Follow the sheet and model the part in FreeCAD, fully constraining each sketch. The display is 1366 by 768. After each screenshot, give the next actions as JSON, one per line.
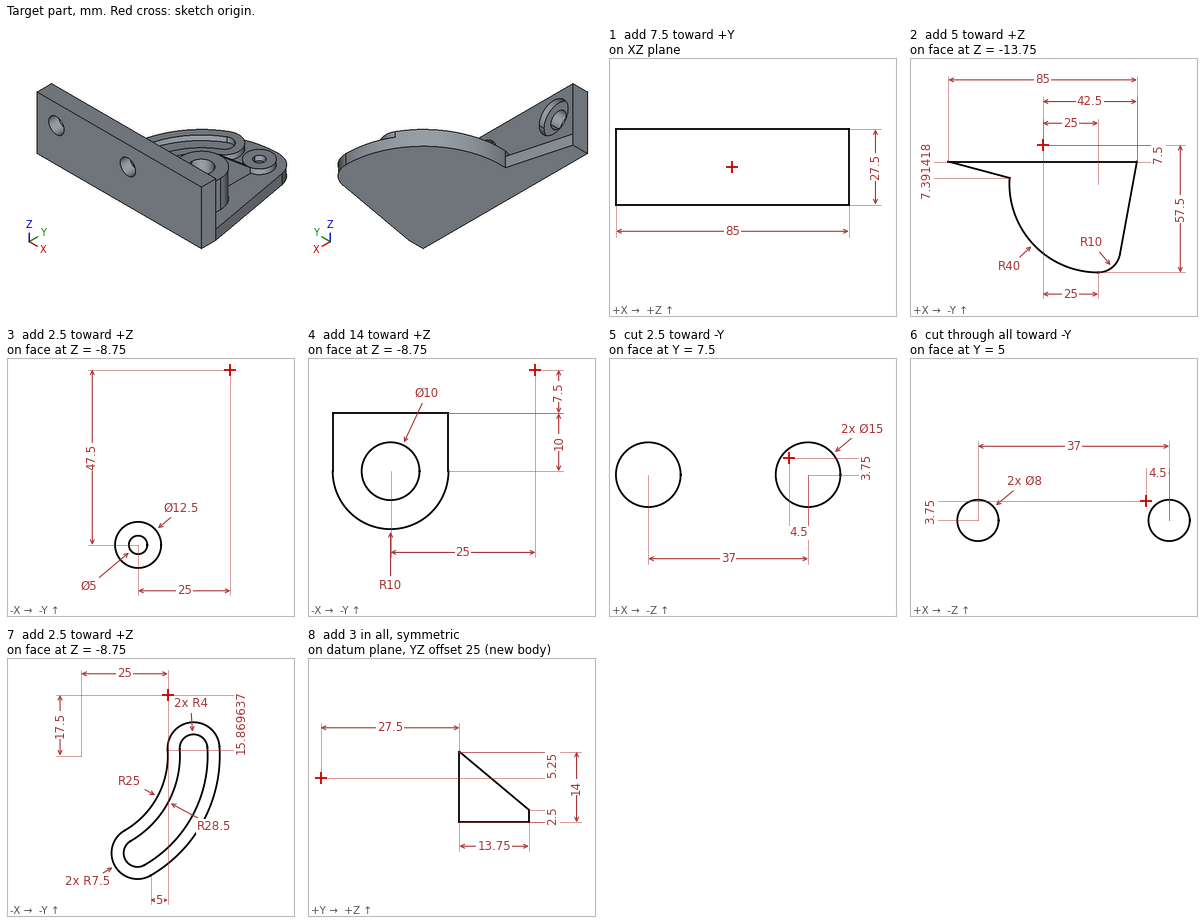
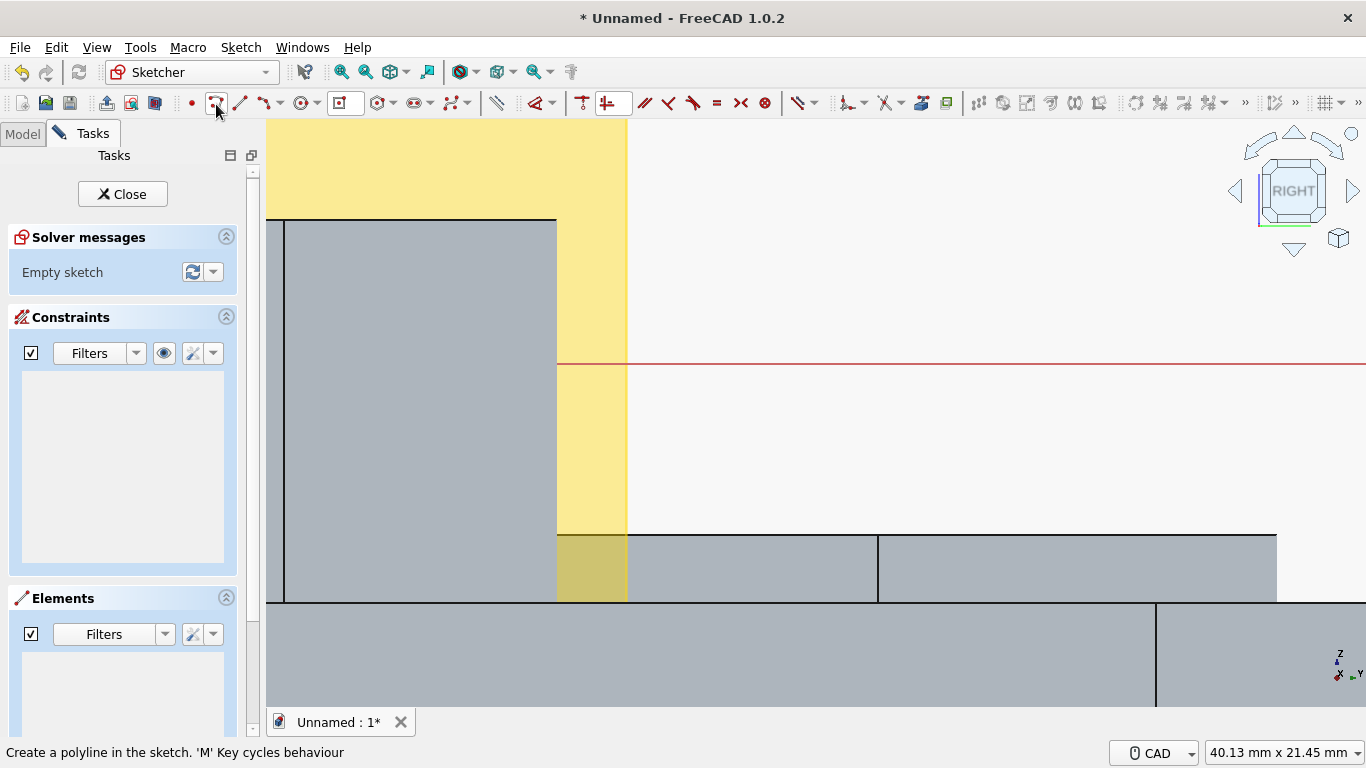
{"action": "left_click", "coordinate": [558, 220]}
{"action": "left_click", "coordinate": [558, 603]}
{"action": "left_click", "coordinate": [935, 603]}
{"action": "left_click", "coordinate": [935, 535]}
{"action": "left_click", "coordinate": [558, 221]}
{"action": "key", "text": "Escape"}
{"action": "key", "text": "Escape"}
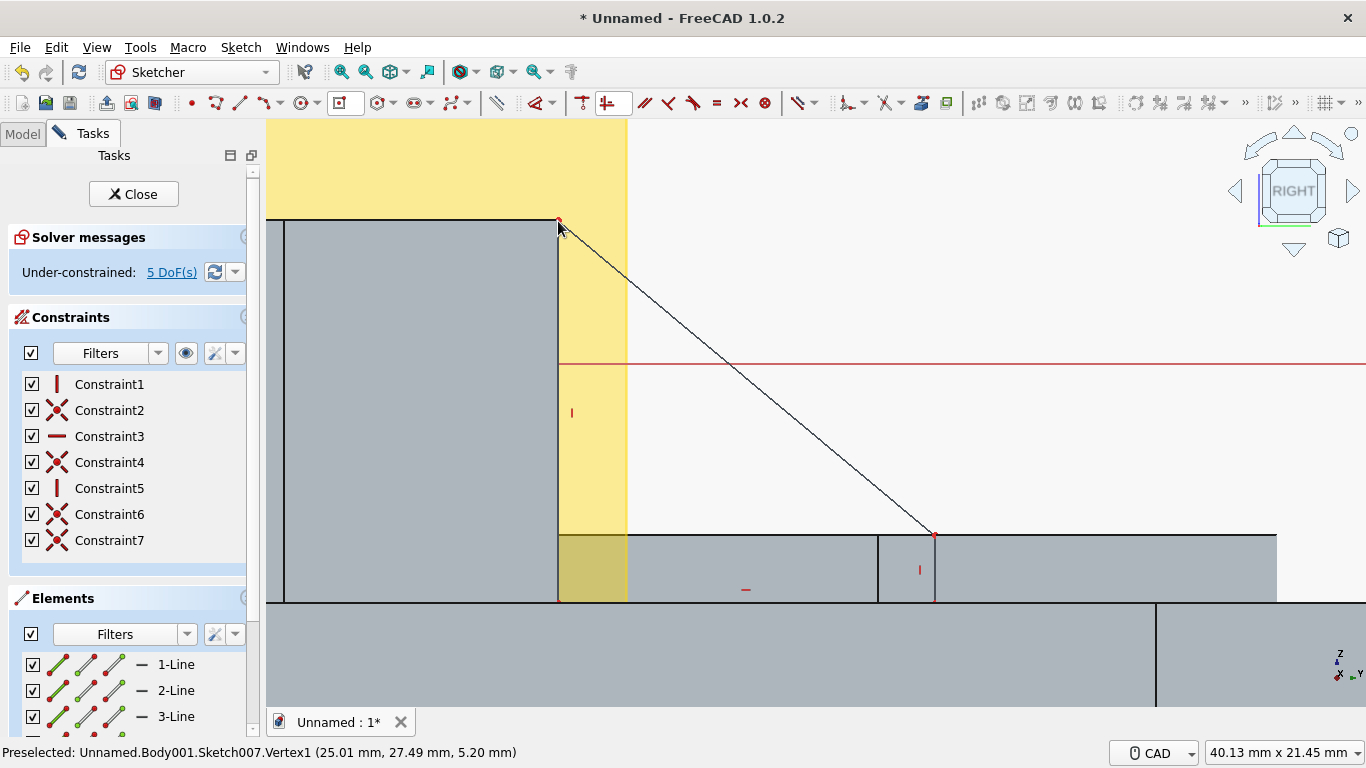
{"action": "left_click", "coordinate": [536, 104]}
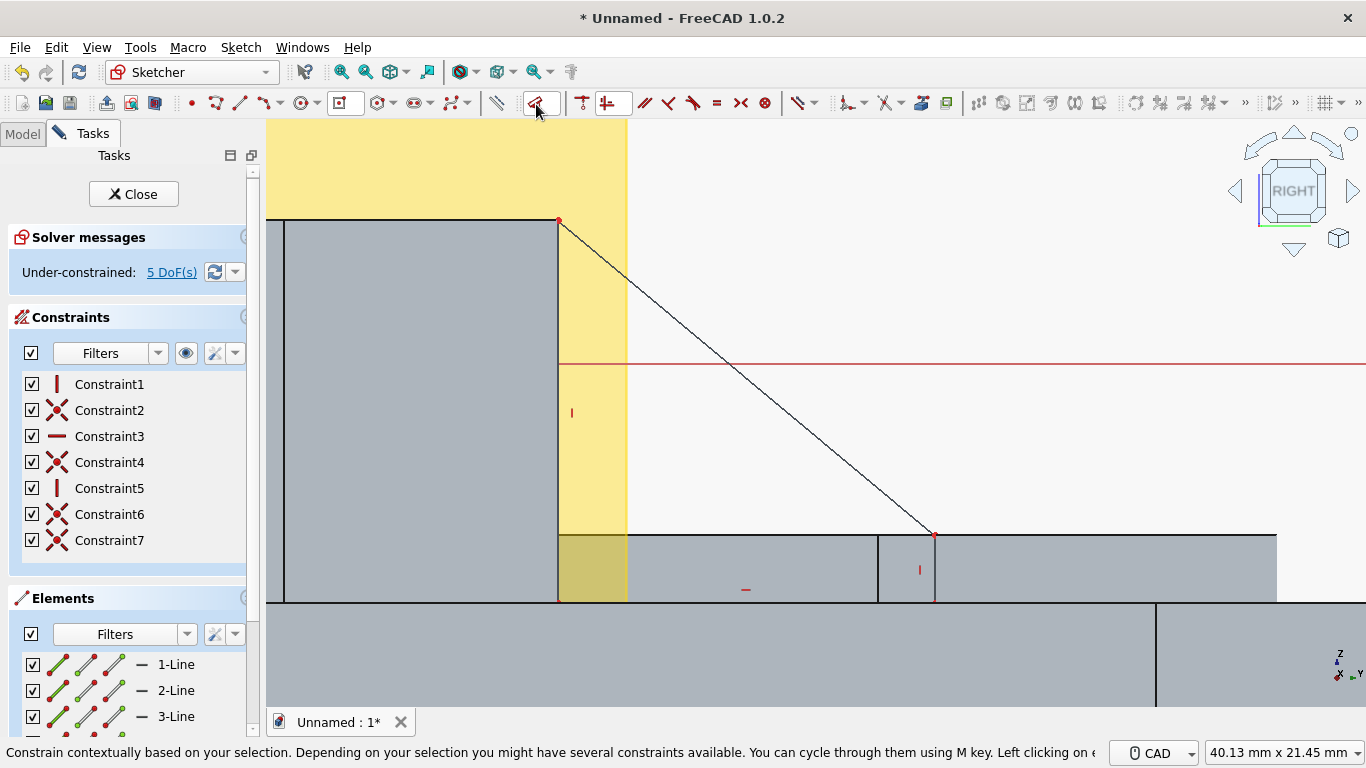
{"action": "left_click", "coordinate": [558, 336]}
{"action": "left_click", "coordinate": [524, 412]}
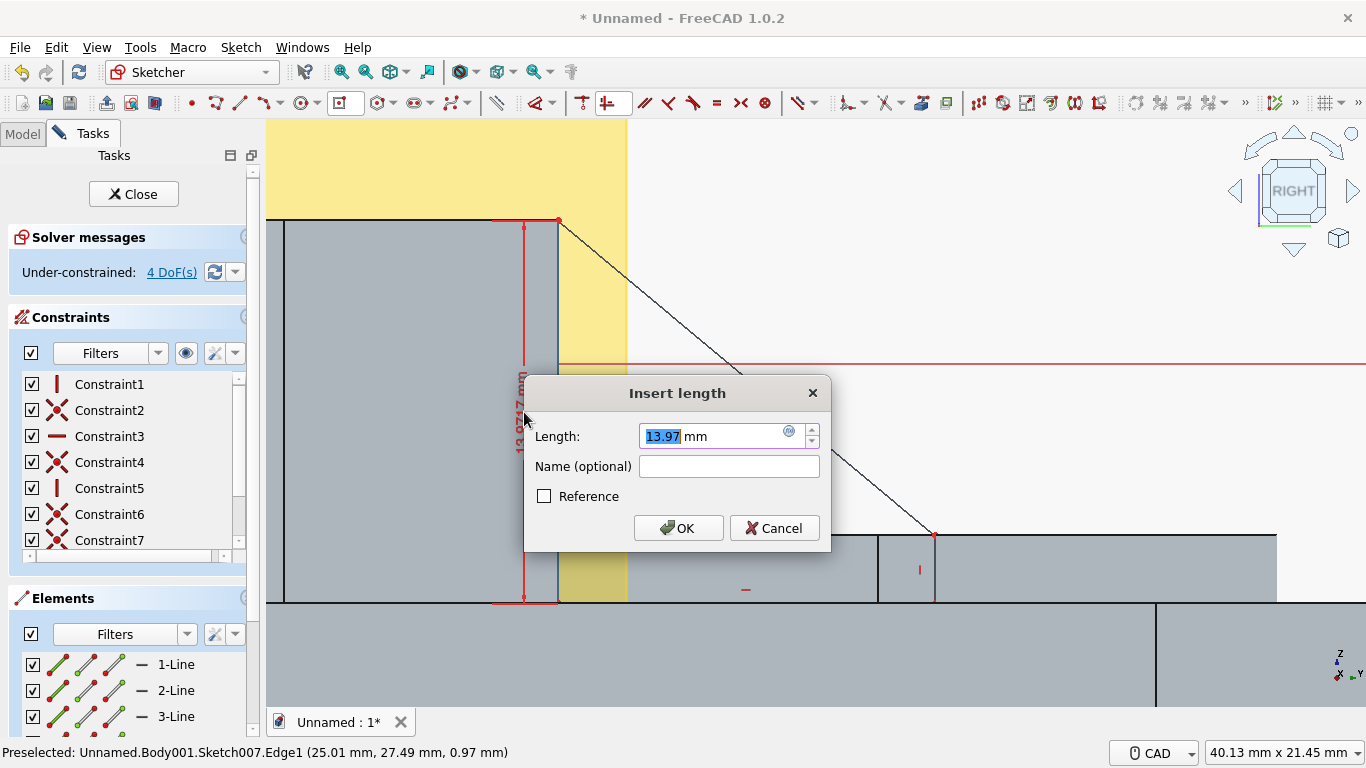
{"action": "type", "text": "14"}
{"action": "key", "text": "Return"}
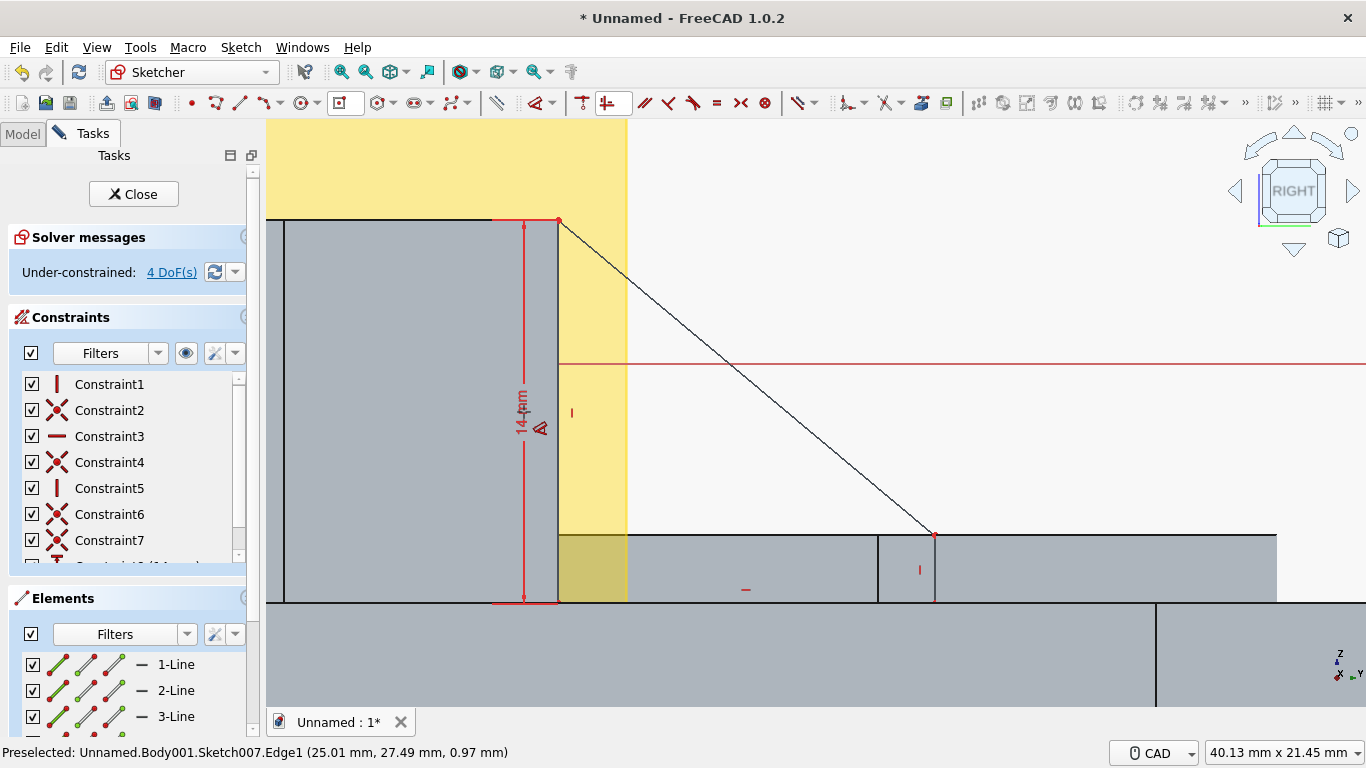
{"action": "left_click", "coordinate": [935, 584]}
{"action": "left_click", "coordinate": [969, 570]}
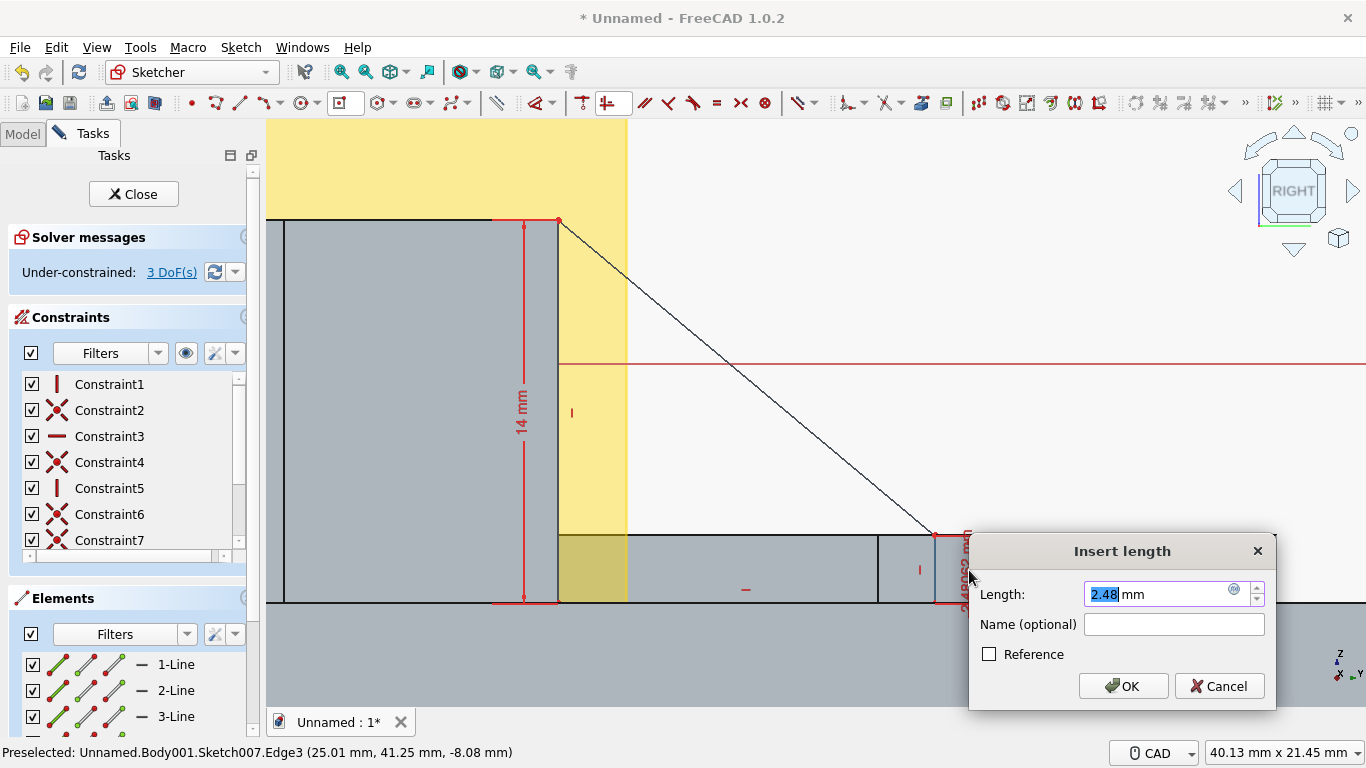
{"action": "type", "text": "2.5"}
{"action": "key", "text": "Return"}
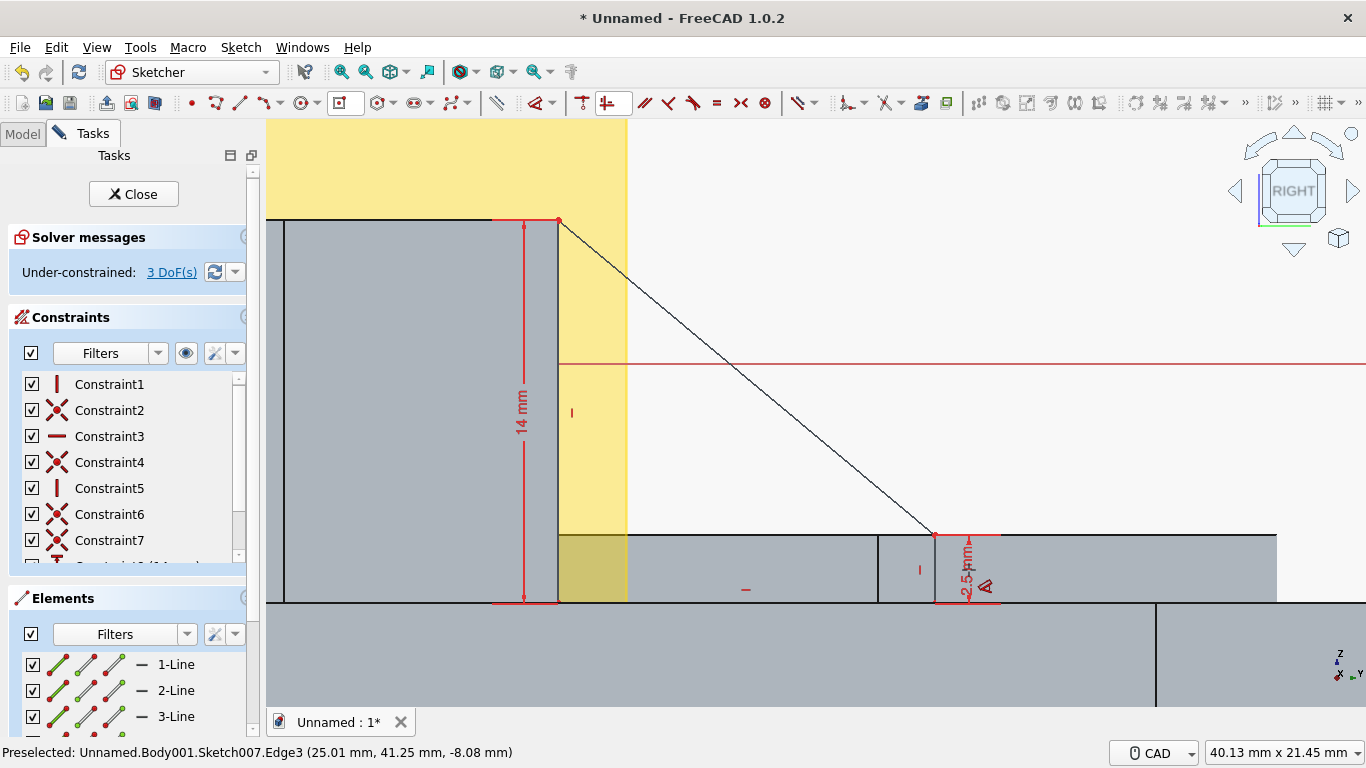
{"action": "left_click", "coordinate": [671, 604]}
{"action": "left_click", "coordinate": [747, 638]}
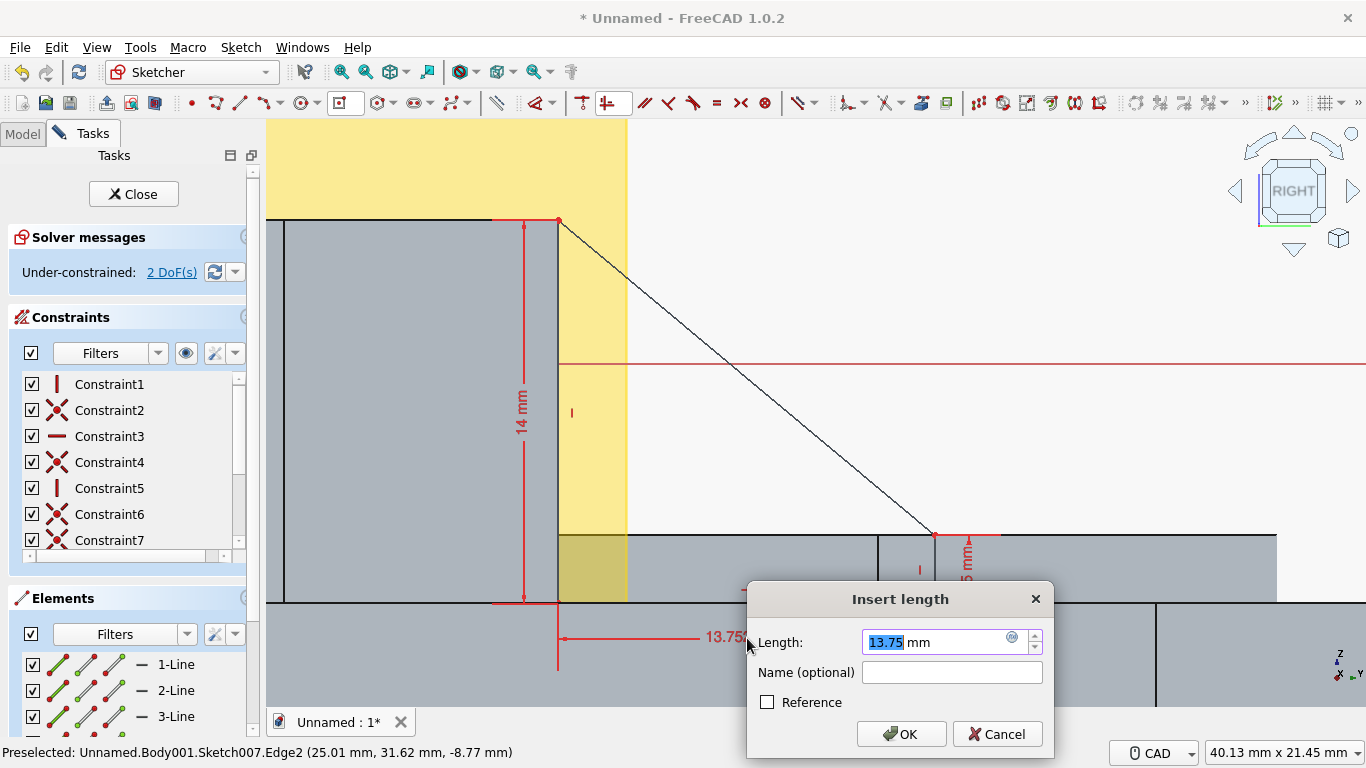
{"action": "type", "text": "13.75"}
{"action": "key", "text": "Return"}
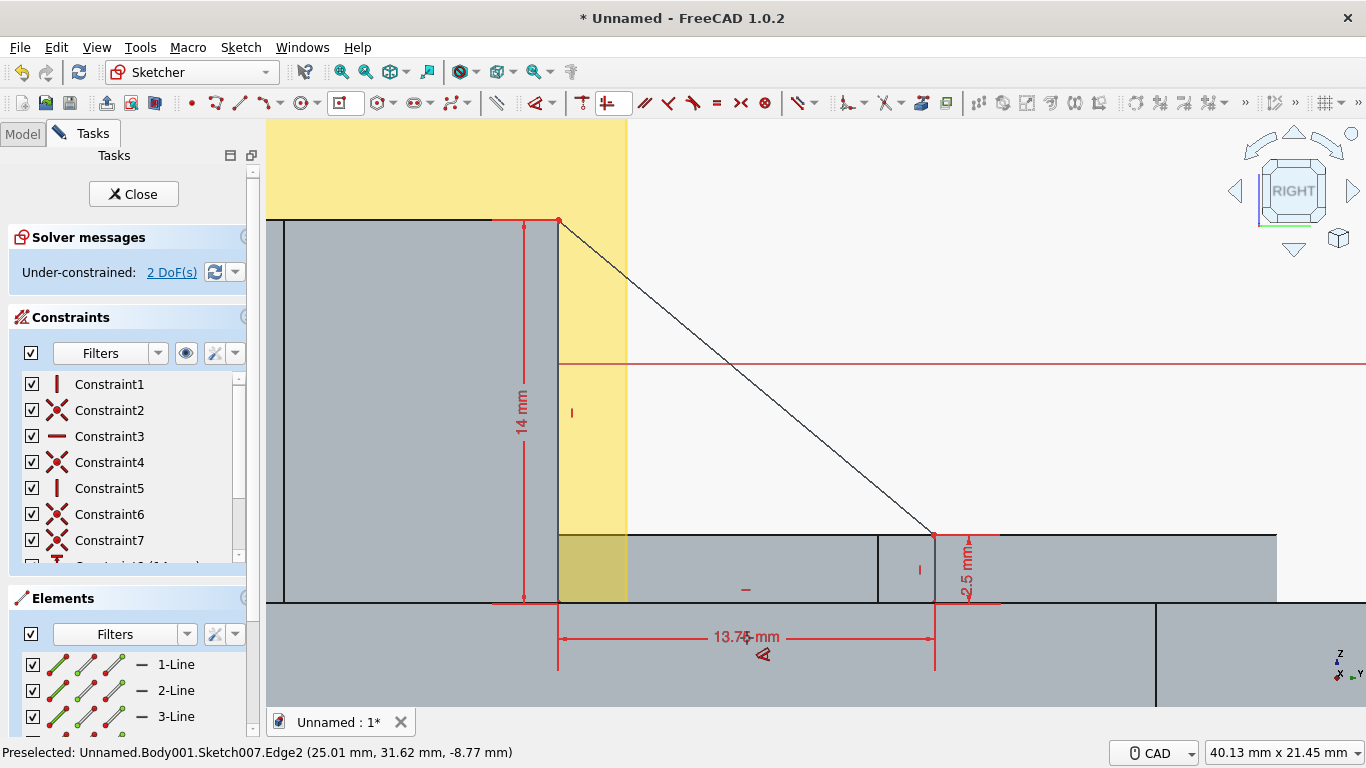
{"action": "left_click", "coordinate": [558, 220]}
{"action": "left_click", "coordinate": [426, 186]}